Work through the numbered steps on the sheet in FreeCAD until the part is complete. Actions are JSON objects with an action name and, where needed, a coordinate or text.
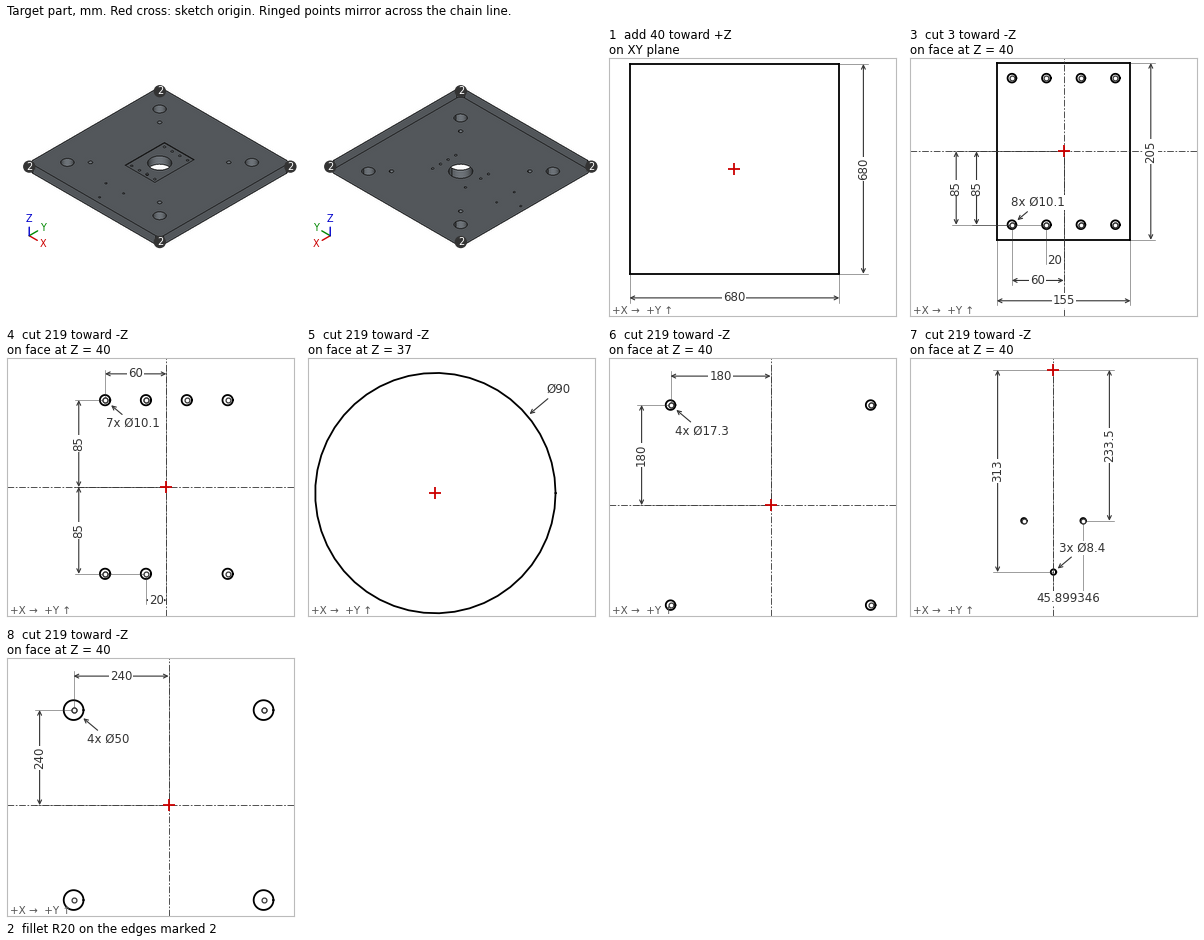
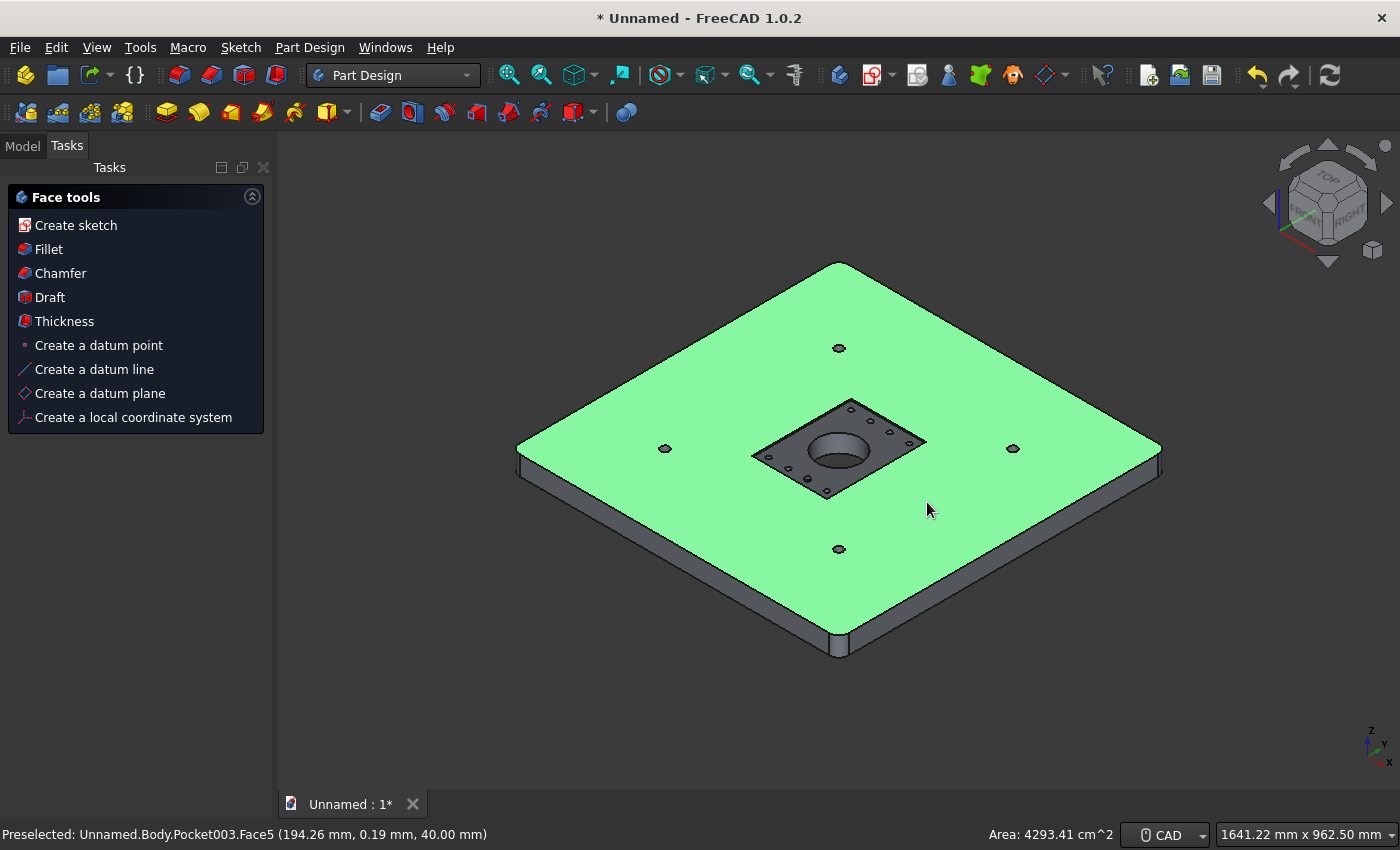
{"action": "left_click", "coordinate": [872, 76]}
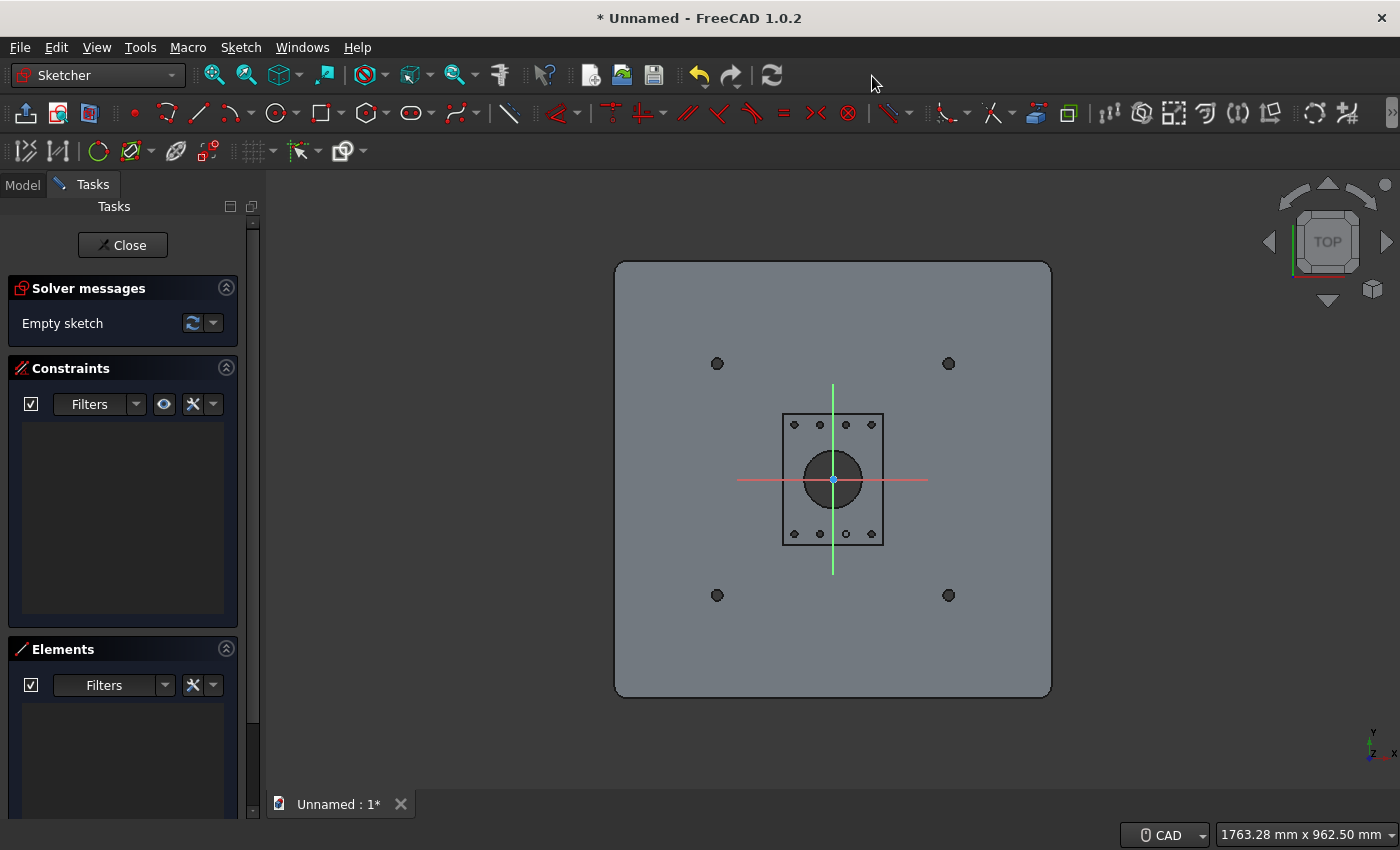
{"action": "scroll", "coordinate": [844, 683], "scroll_direction": "up", "scroll_amount": 10}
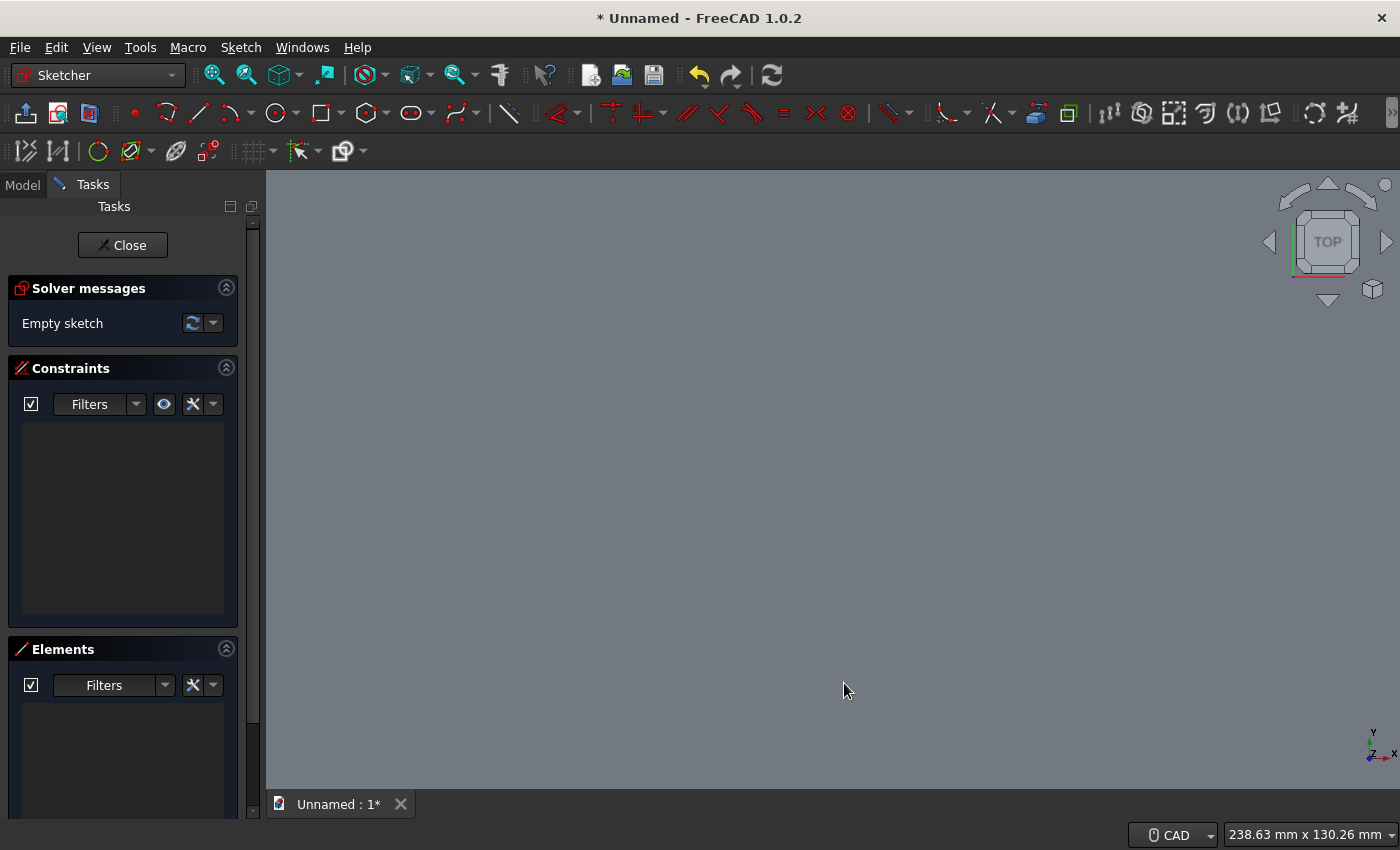
{"action": "left_click", "coordinate": [276, 114]}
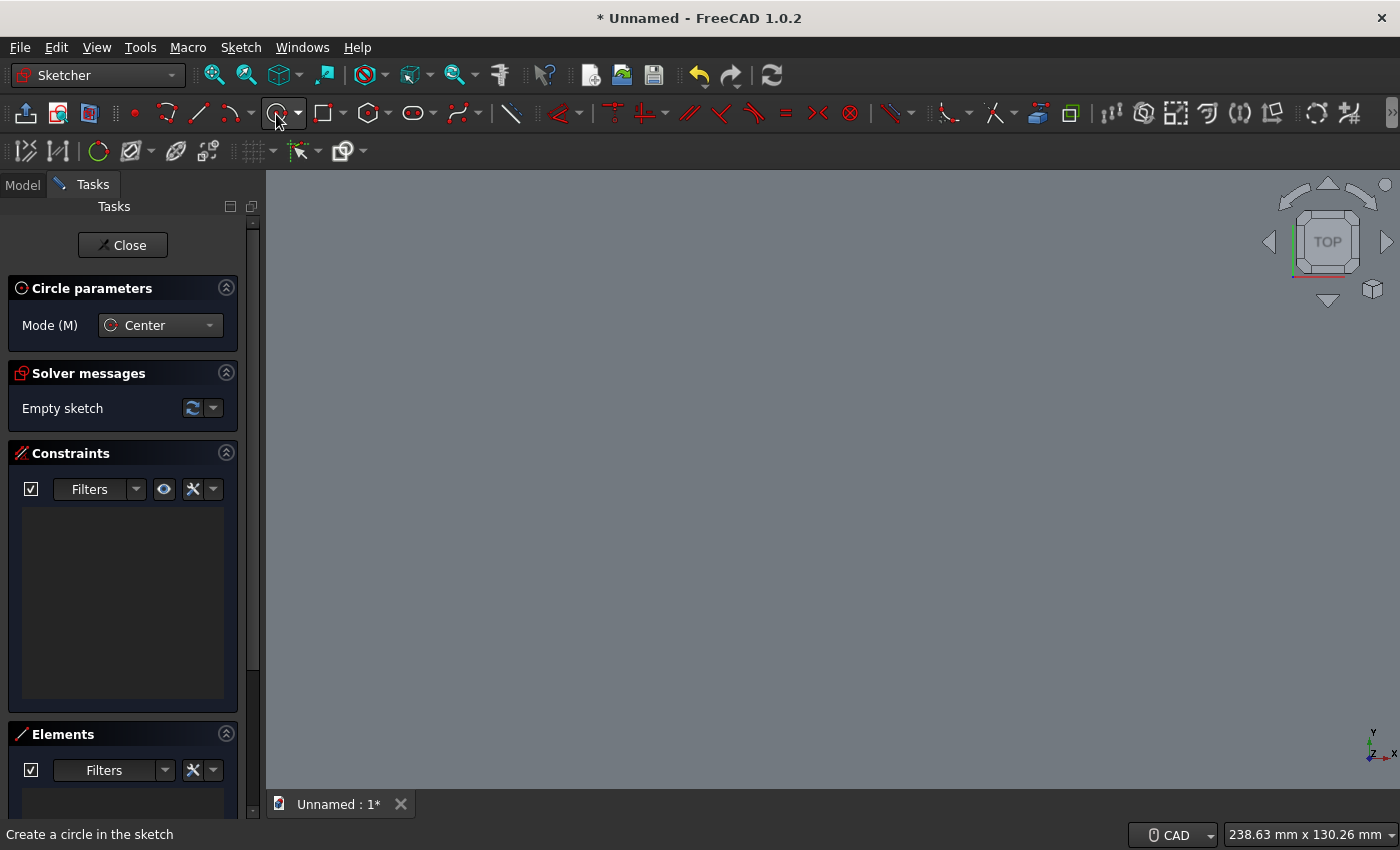
{"action": "left_click", "coordinate": [759, 661]}
{"action": "left_click", "coordinate": [774, 647]}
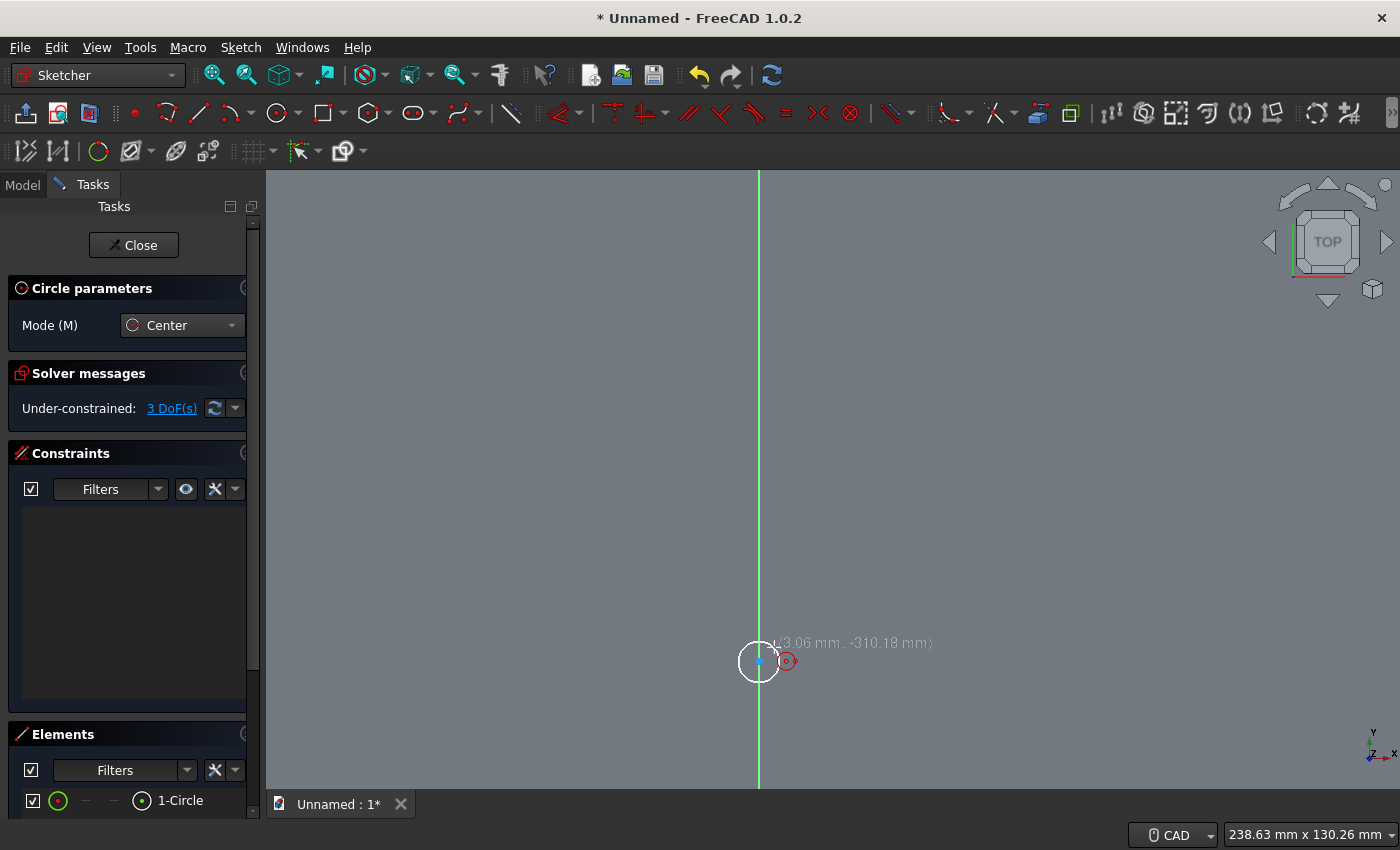
{"action": "left_click", "coordinate": [978, 284]}
{"action": "left_click", "coordinate": [992, 270]}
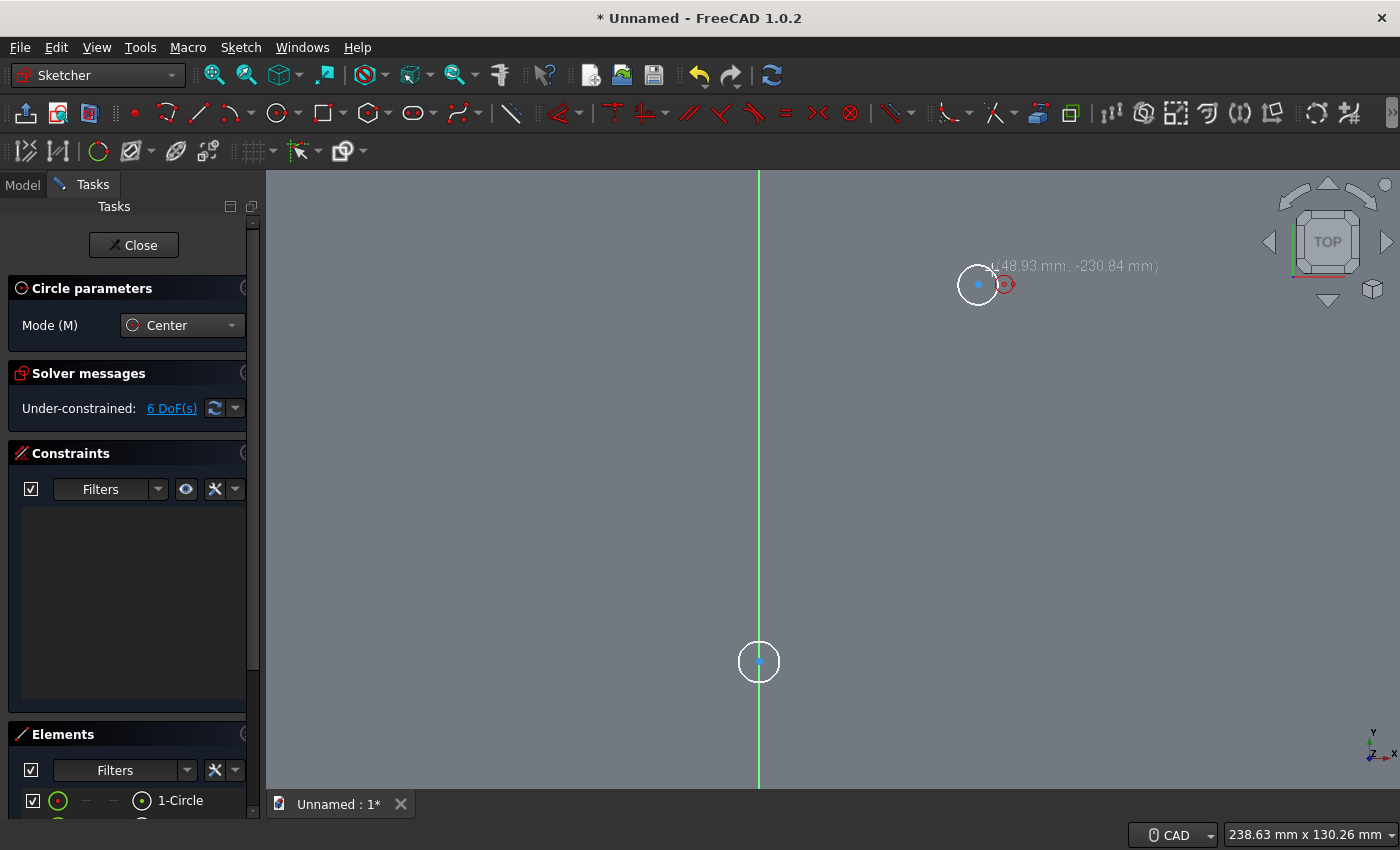
{"action": "left_click", "coordinate": [541, 284]}
{"action": "left_click", "coordinate": [555, 270]}
{"action": "key", "text": "Escape"}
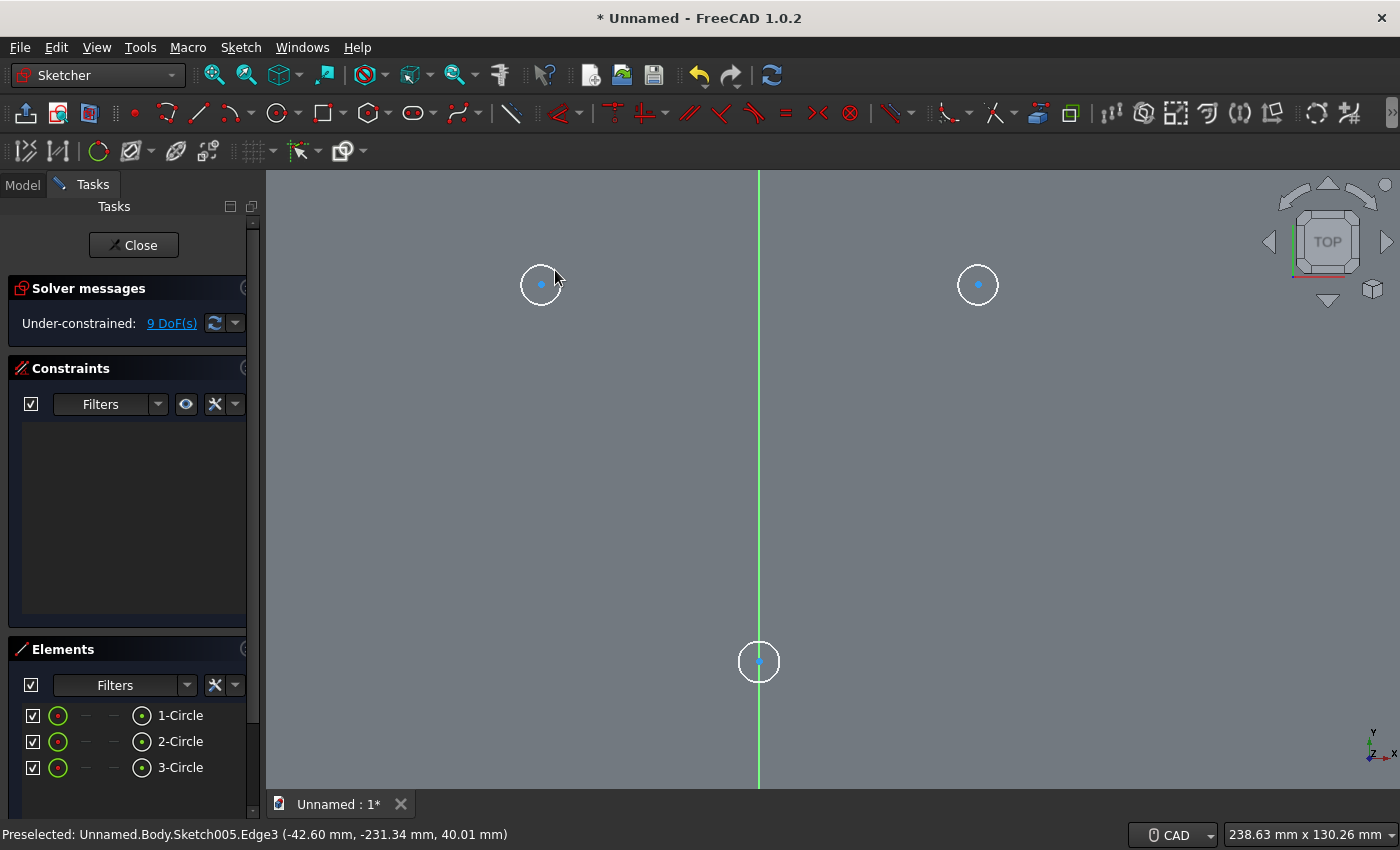
{"action": "left_click", "coordinate": [773, 647]}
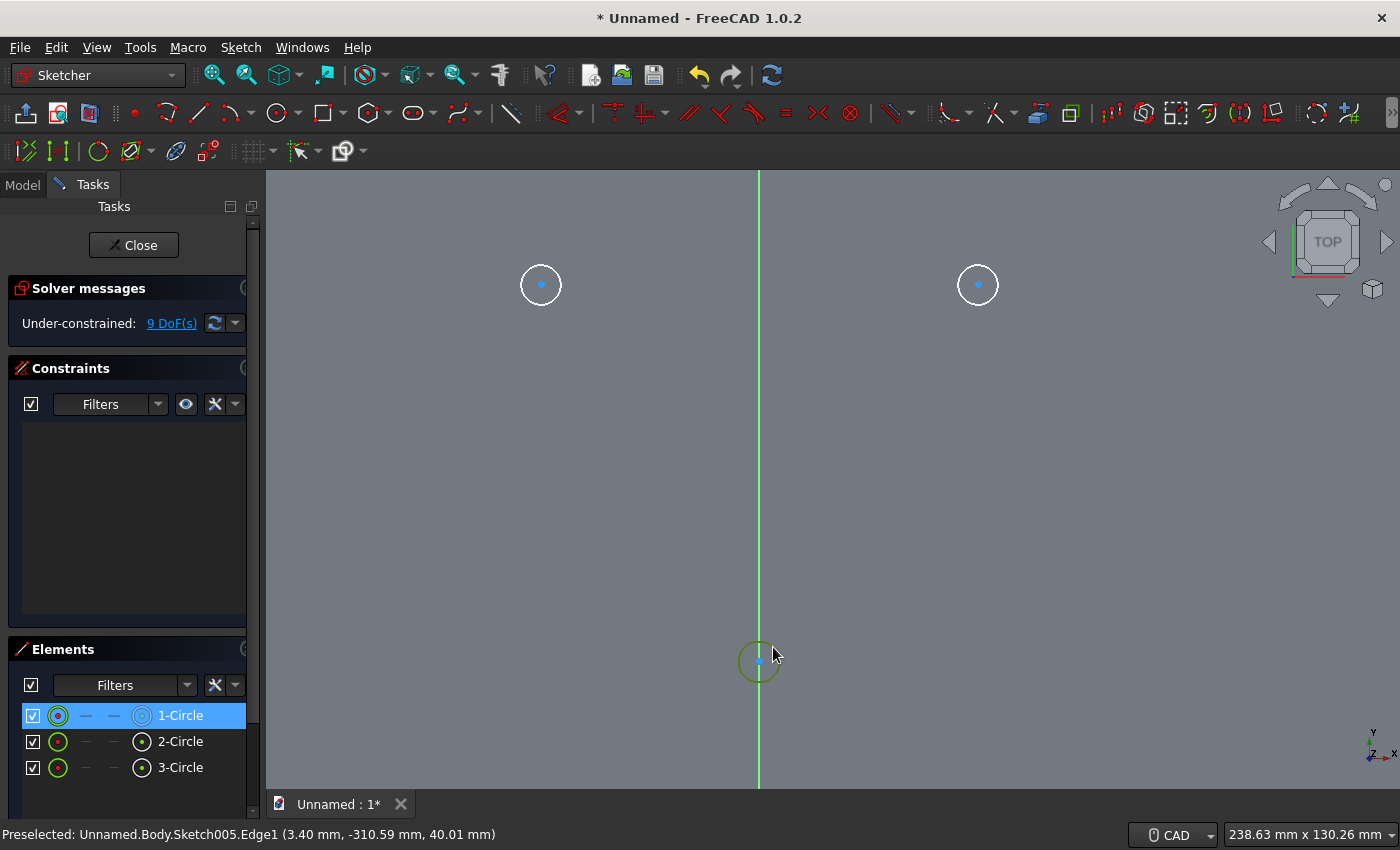
{"action": "left_click", "coordinate": [992, 271]}